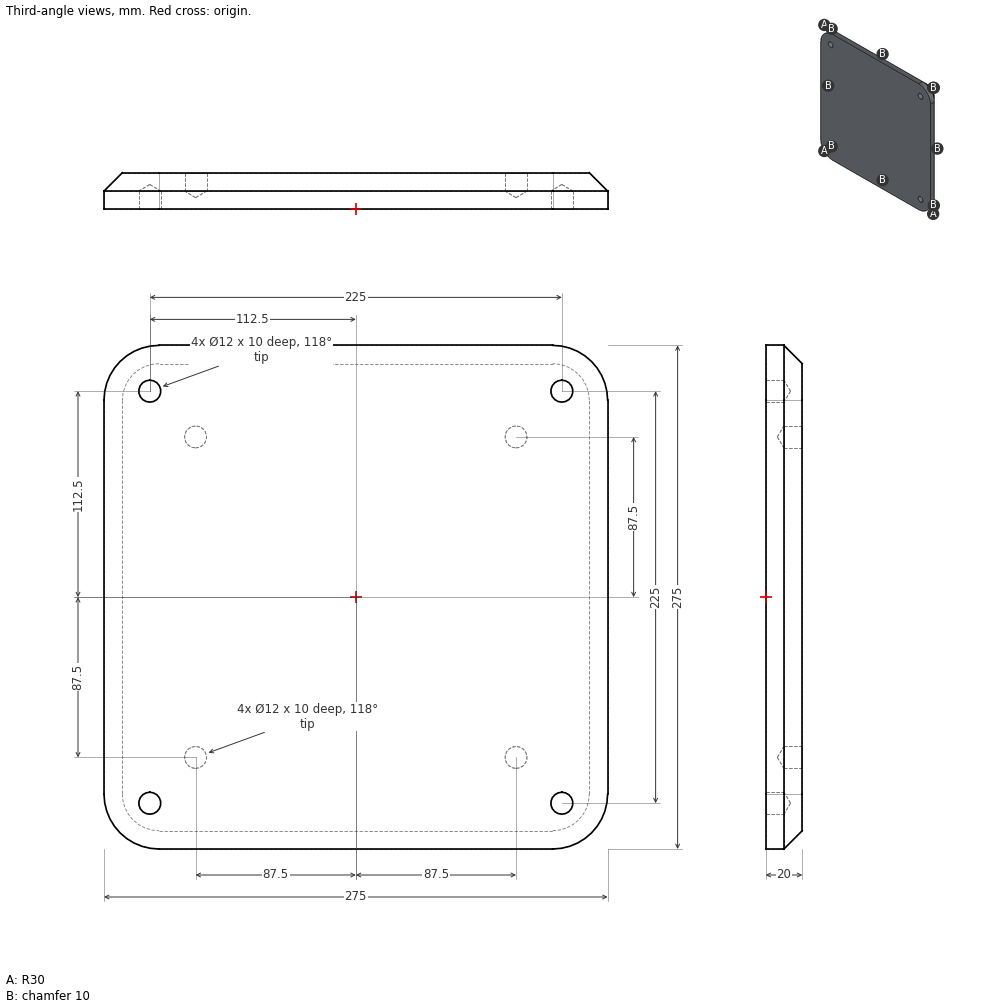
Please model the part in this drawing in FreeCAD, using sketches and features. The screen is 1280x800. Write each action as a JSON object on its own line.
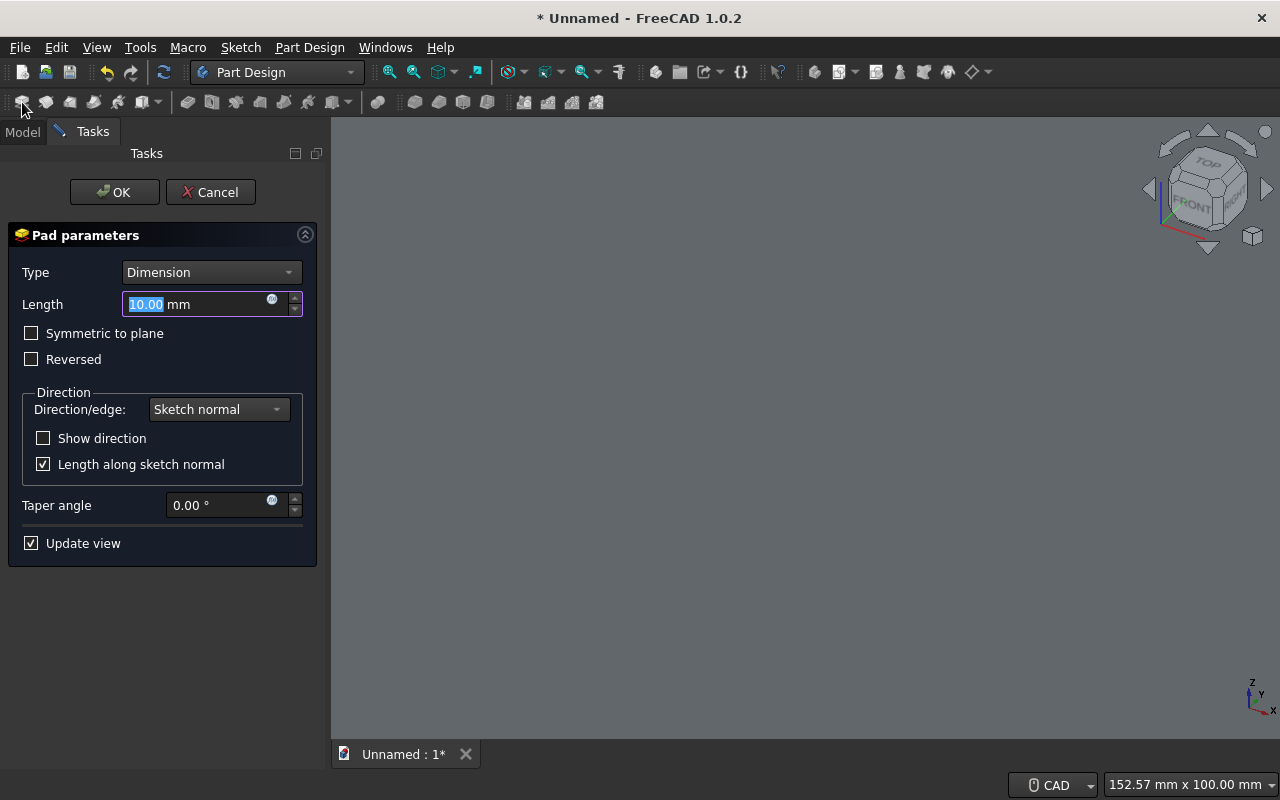
{"action": "type", "text": "20"}
{"action": "key", "text": "Tab"}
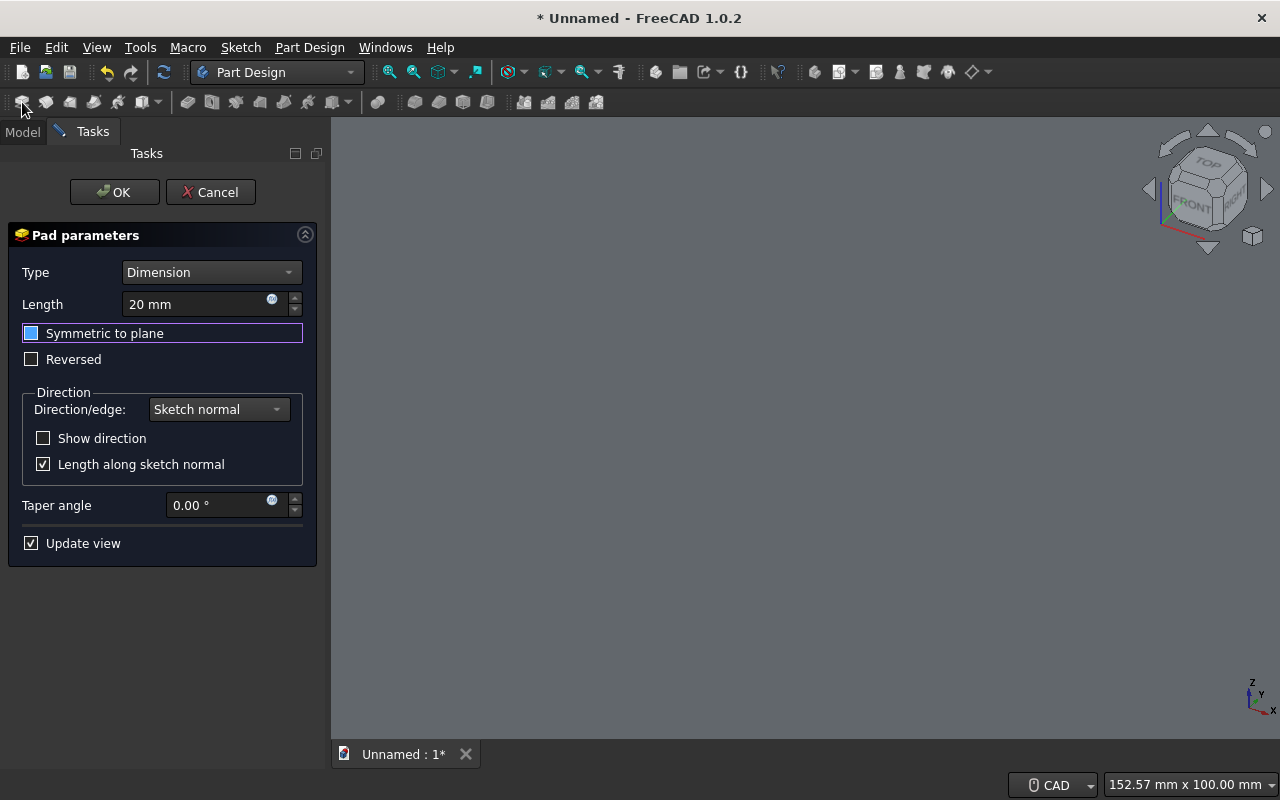
{"action": "left_click", "coordinate": [30, 359]}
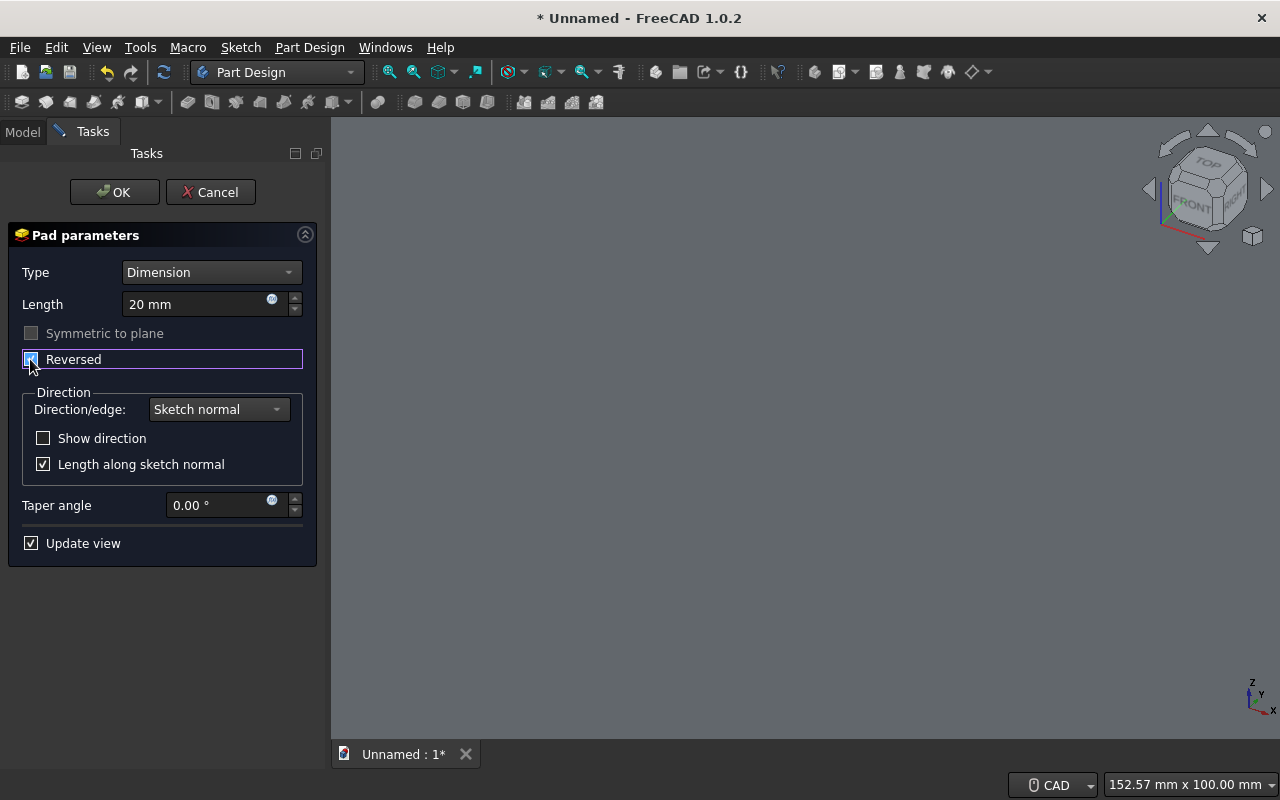
{"action": "left_click", "coordinate": [115, 192]}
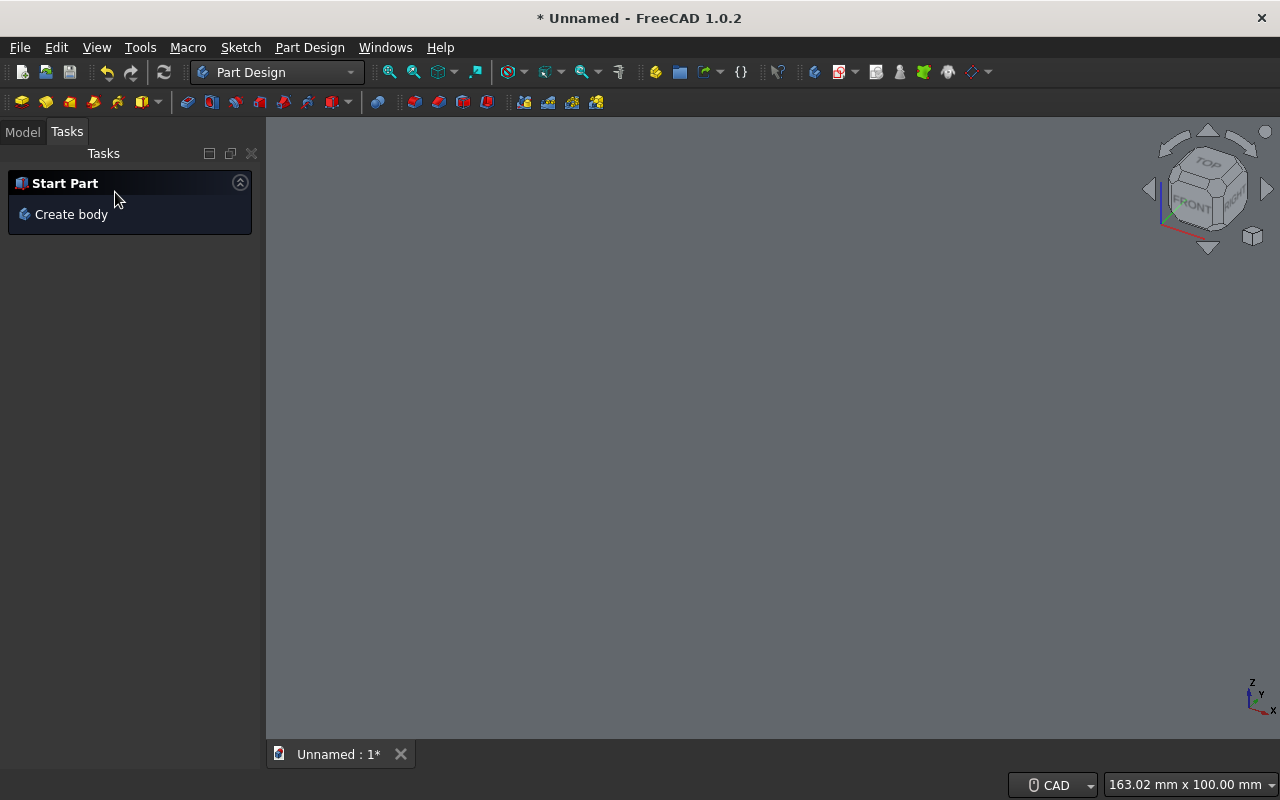
{"action": "key", "text": "v f"}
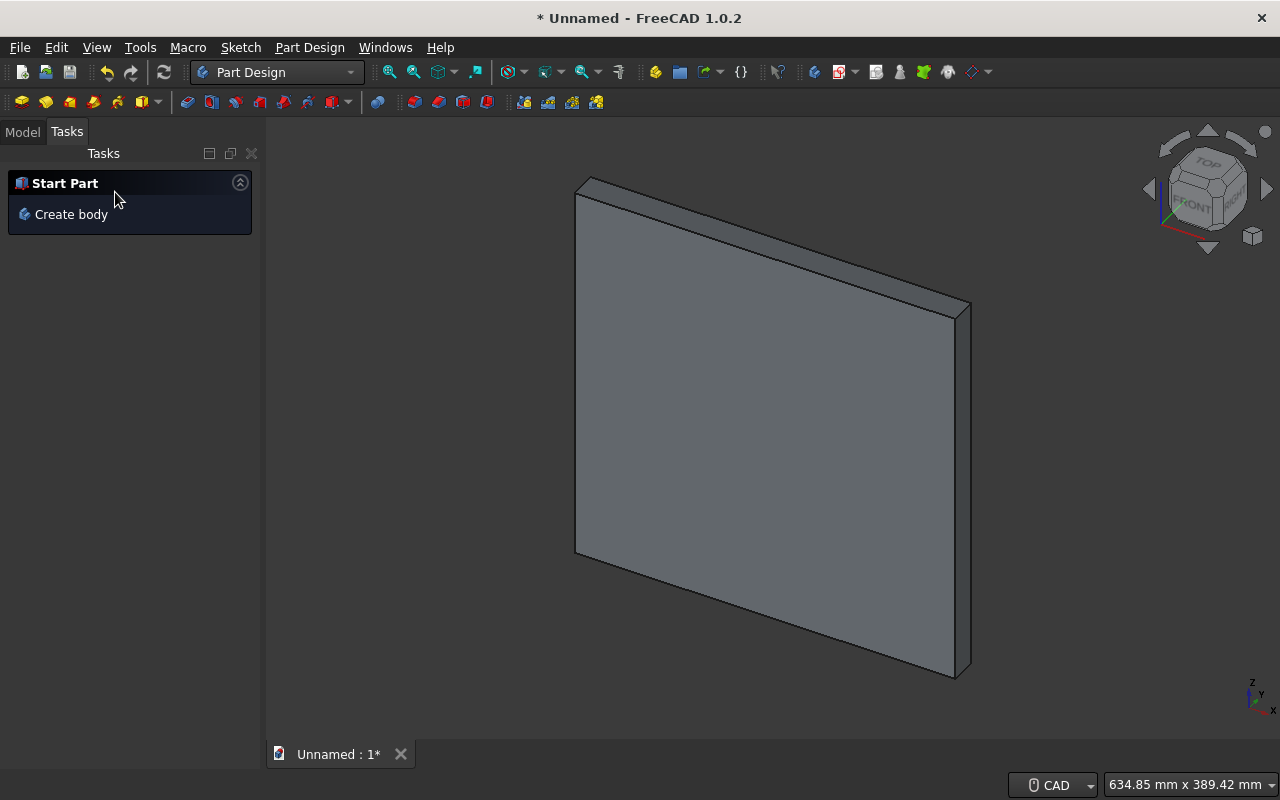
{"action": "left_click", "coordinate": [963, 310]}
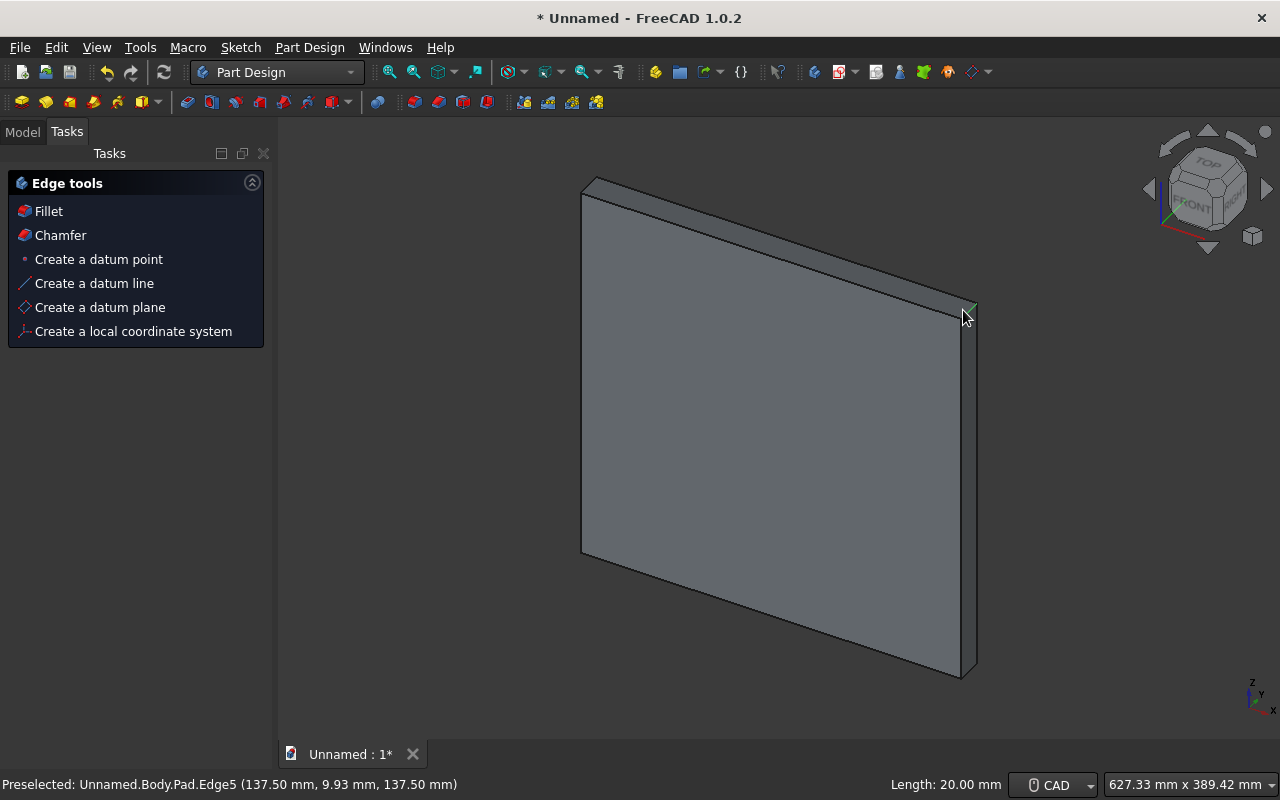
{"action": "key", "text": "0"}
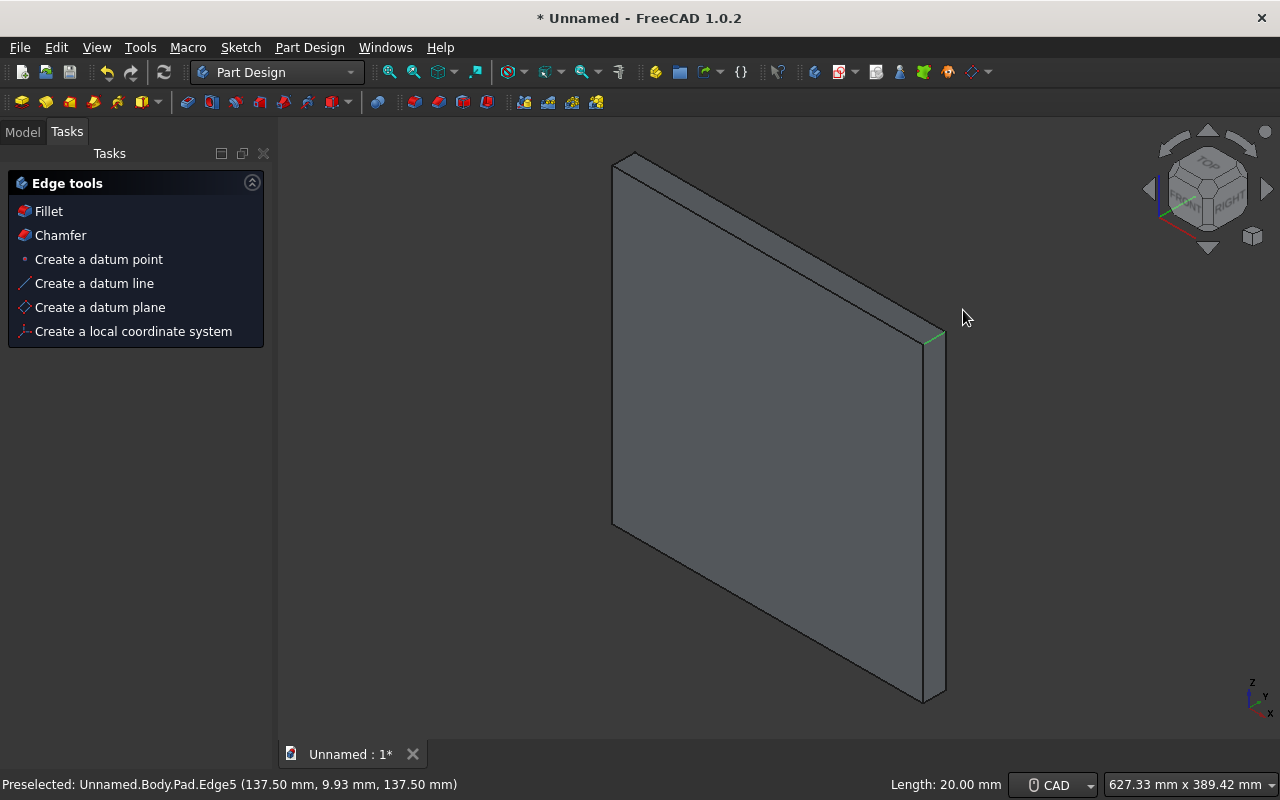
{"action": "key", "text": "2"}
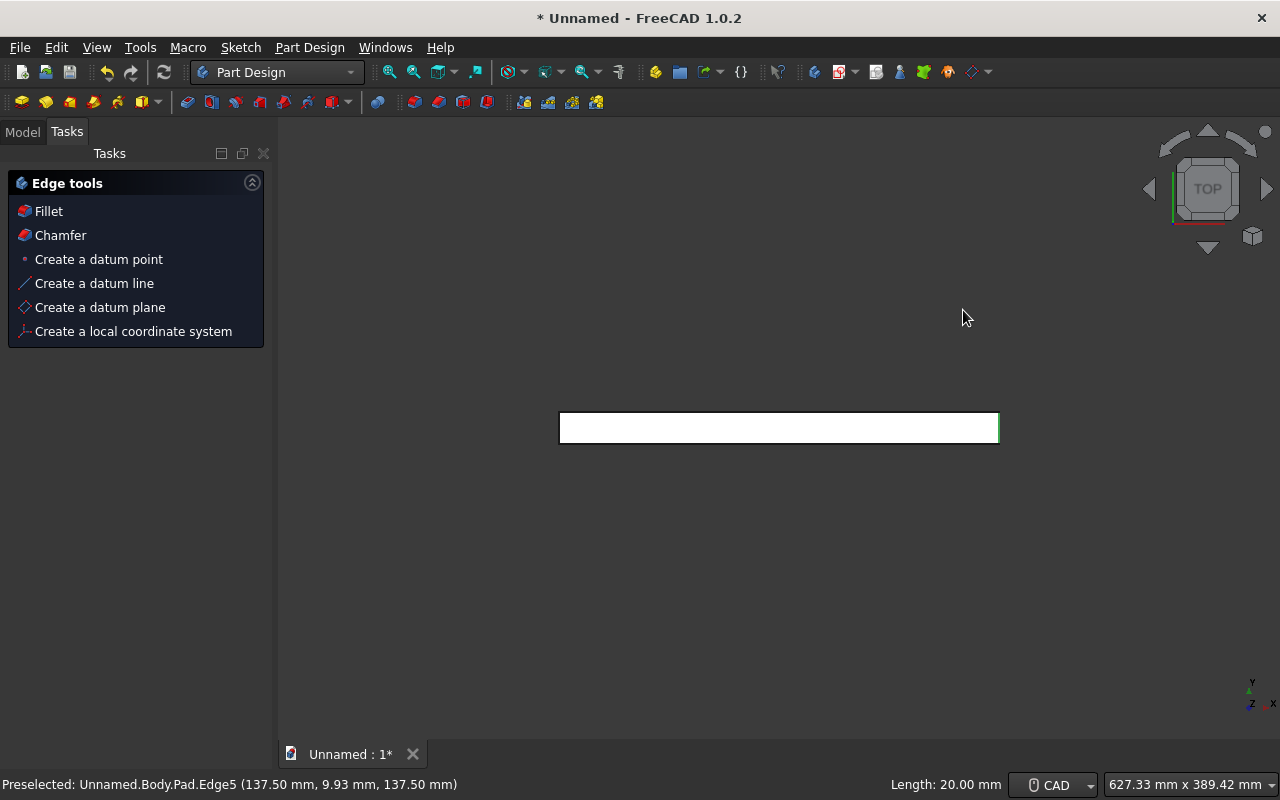
{"action": "key", "text": "v f"}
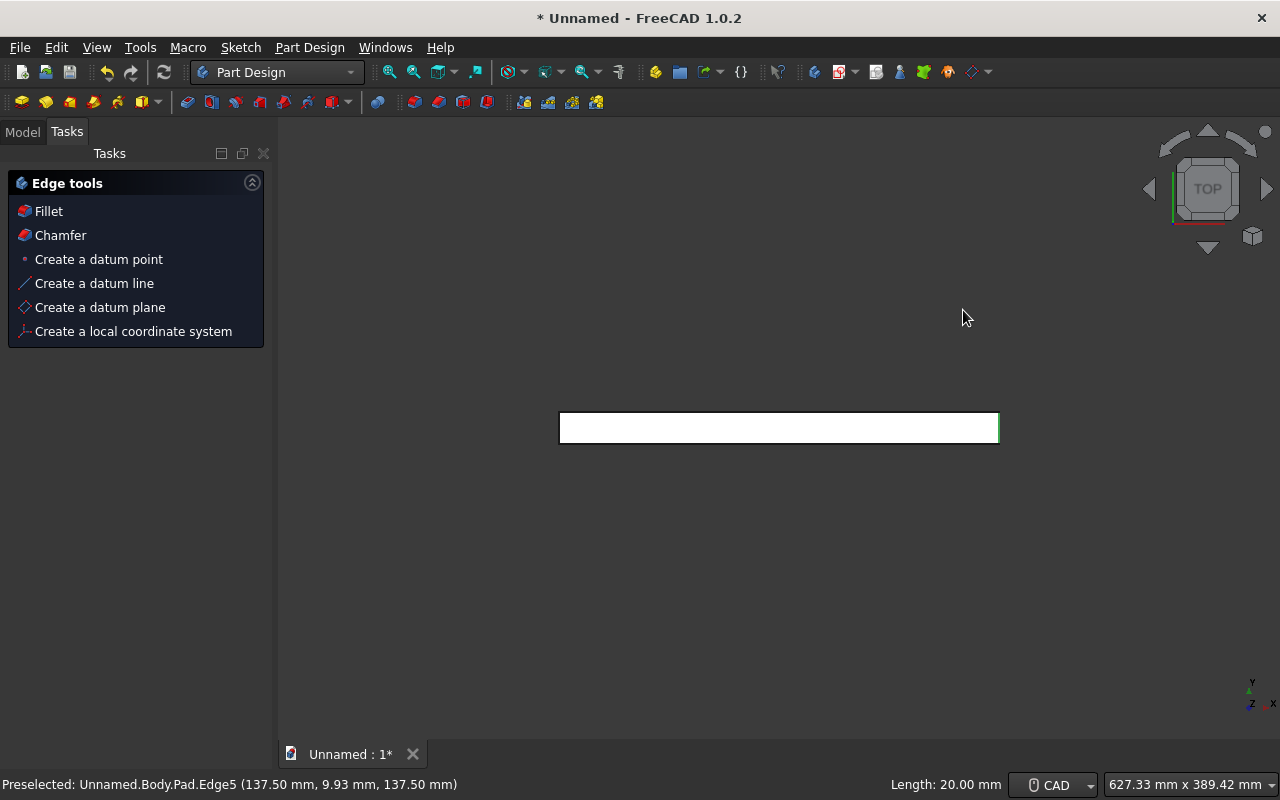
{"action": "left_click", "coordinate": [559, 427], "text": "ctrl"}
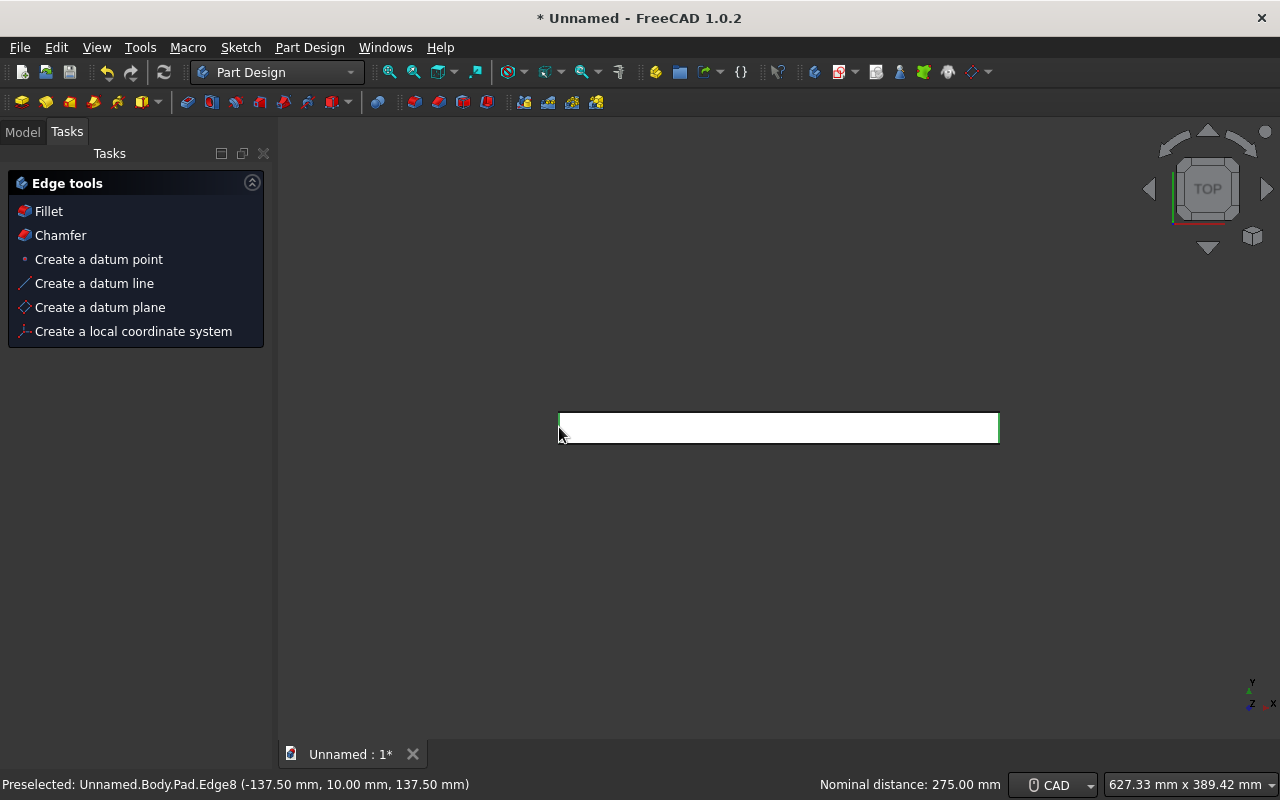
{"action": "key", "text": "1"}